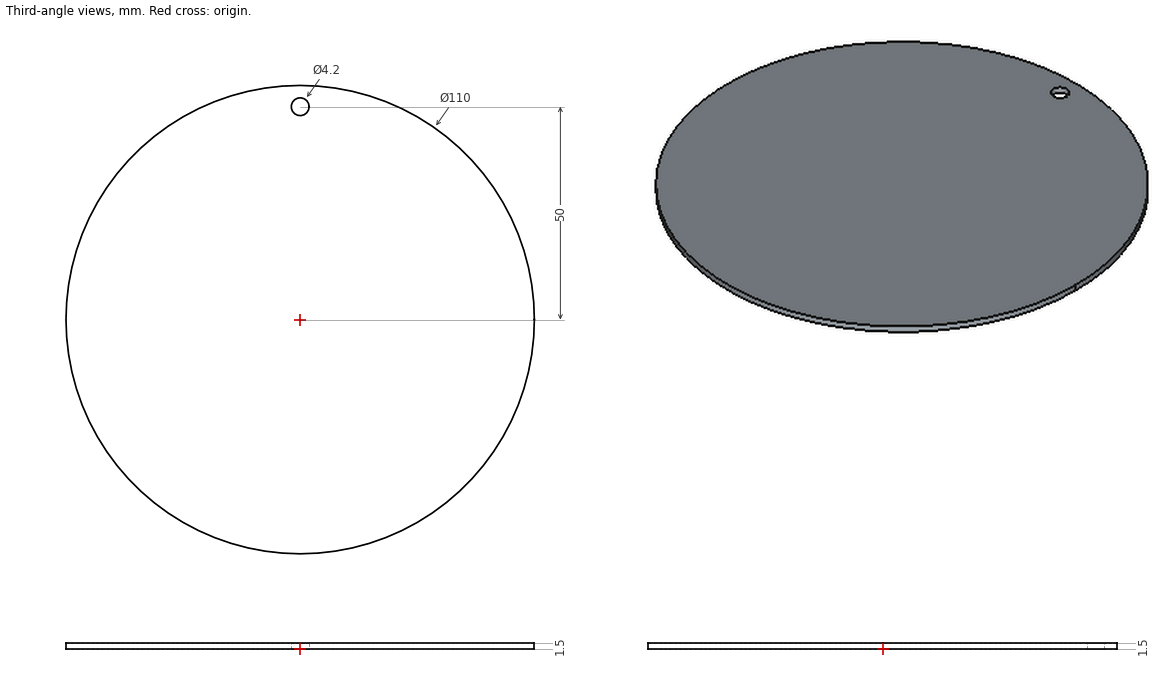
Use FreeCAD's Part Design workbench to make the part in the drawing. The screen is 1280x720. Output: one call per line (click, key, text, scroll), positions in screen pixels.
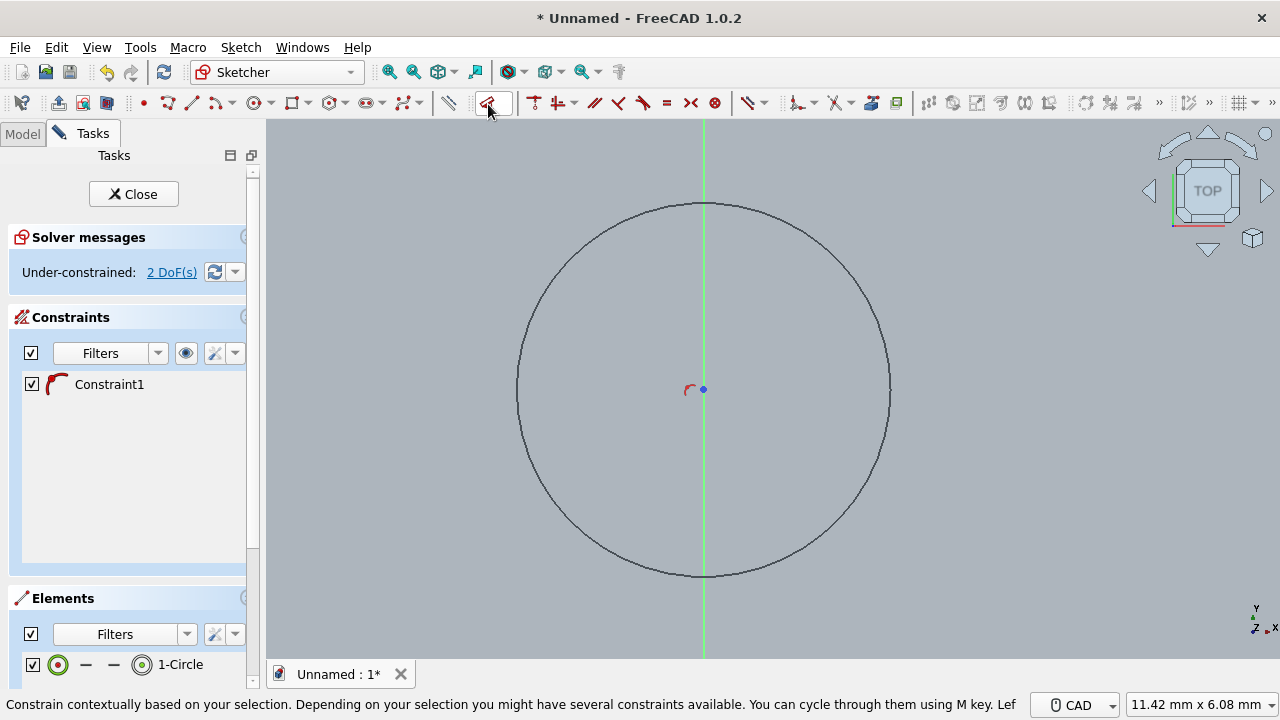
click(835, 257)
click(857, 234)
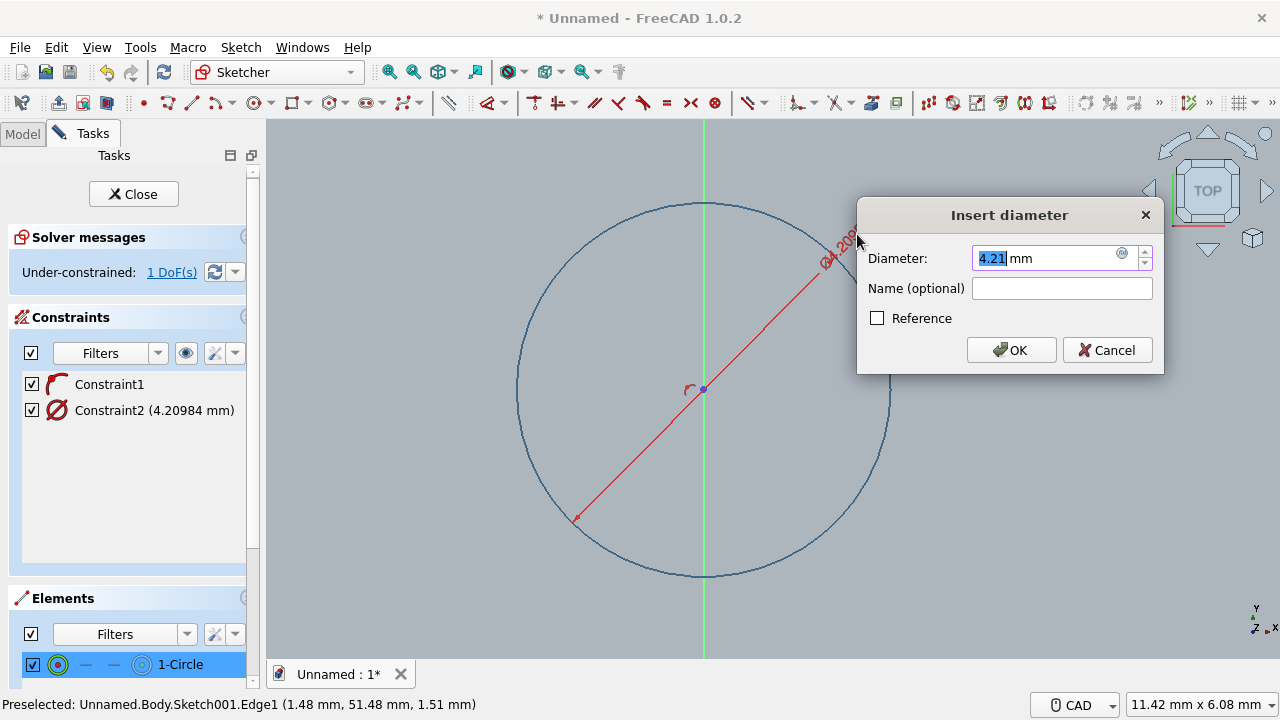
text(4.2)
key(Return)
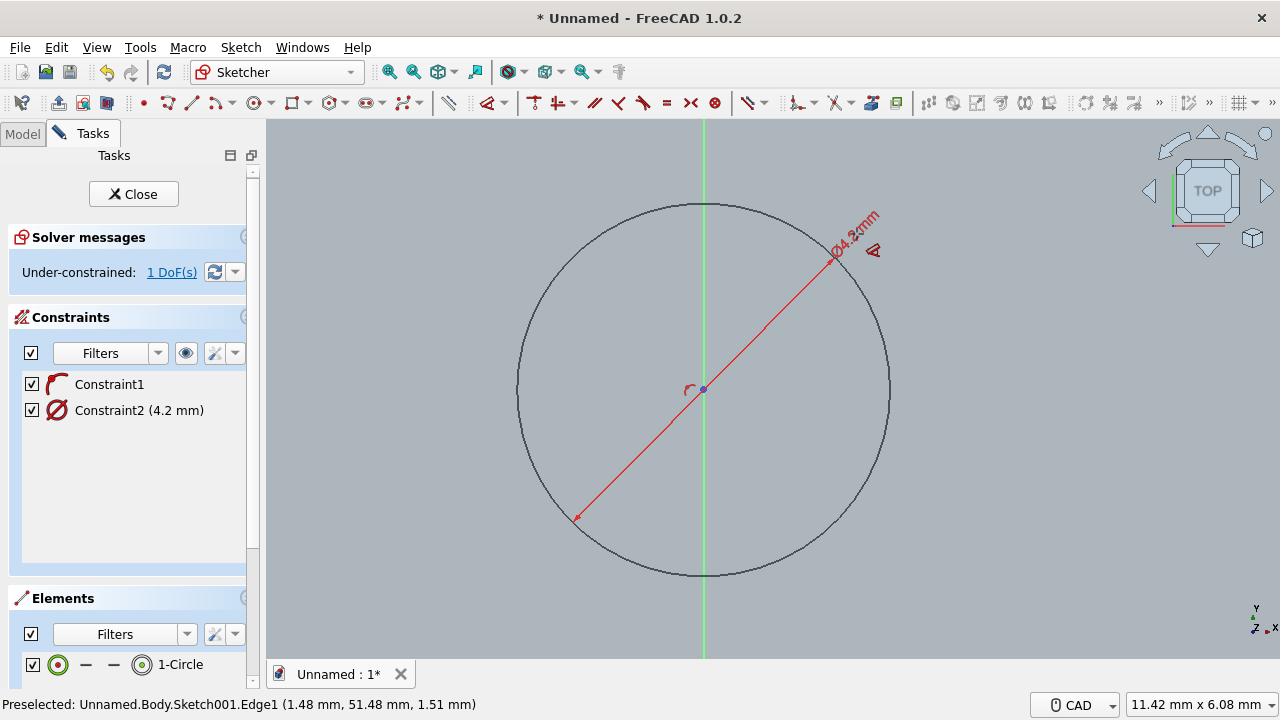
click(704, 390)
click(738, 510)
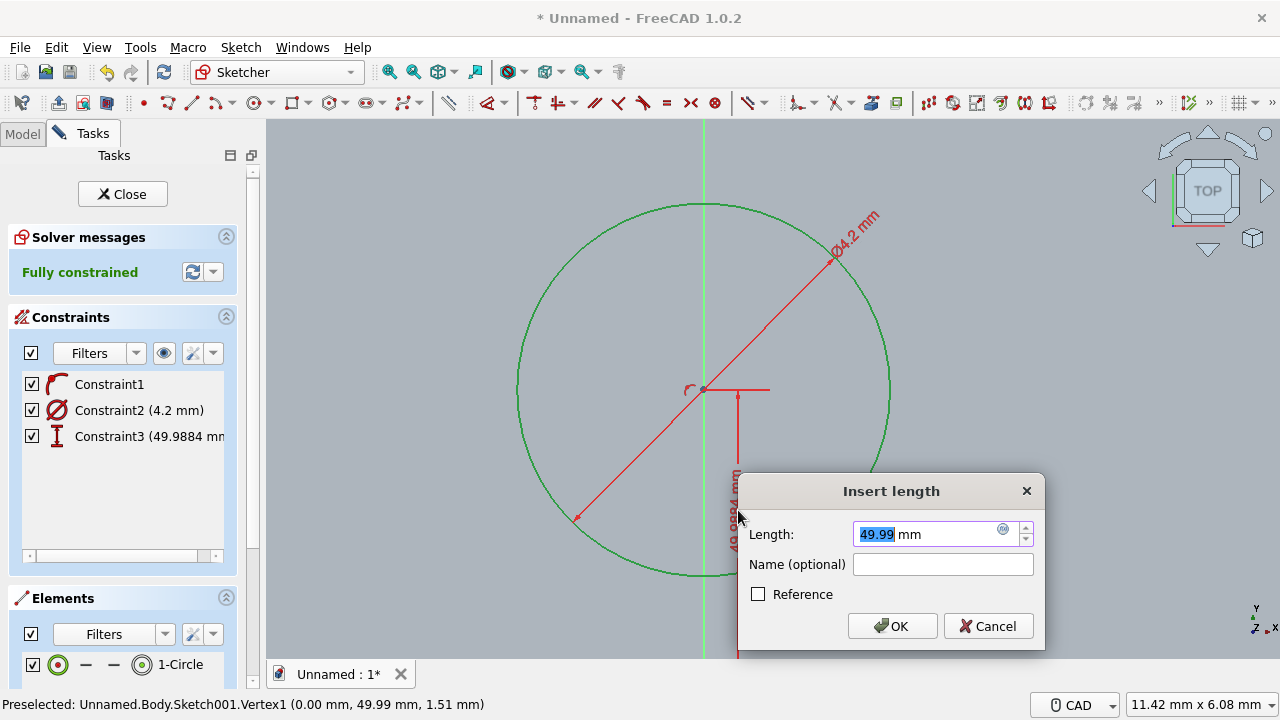
text(50)
key(Return)
key(Escape)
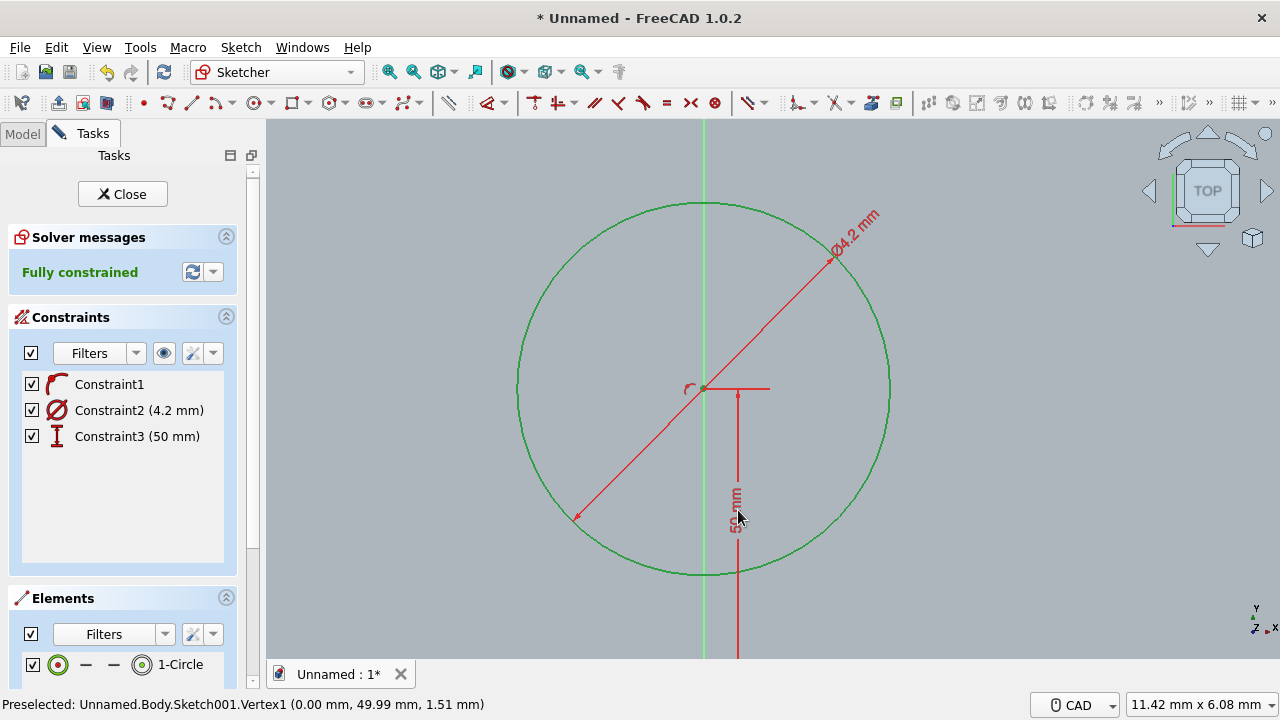
click(123, 194)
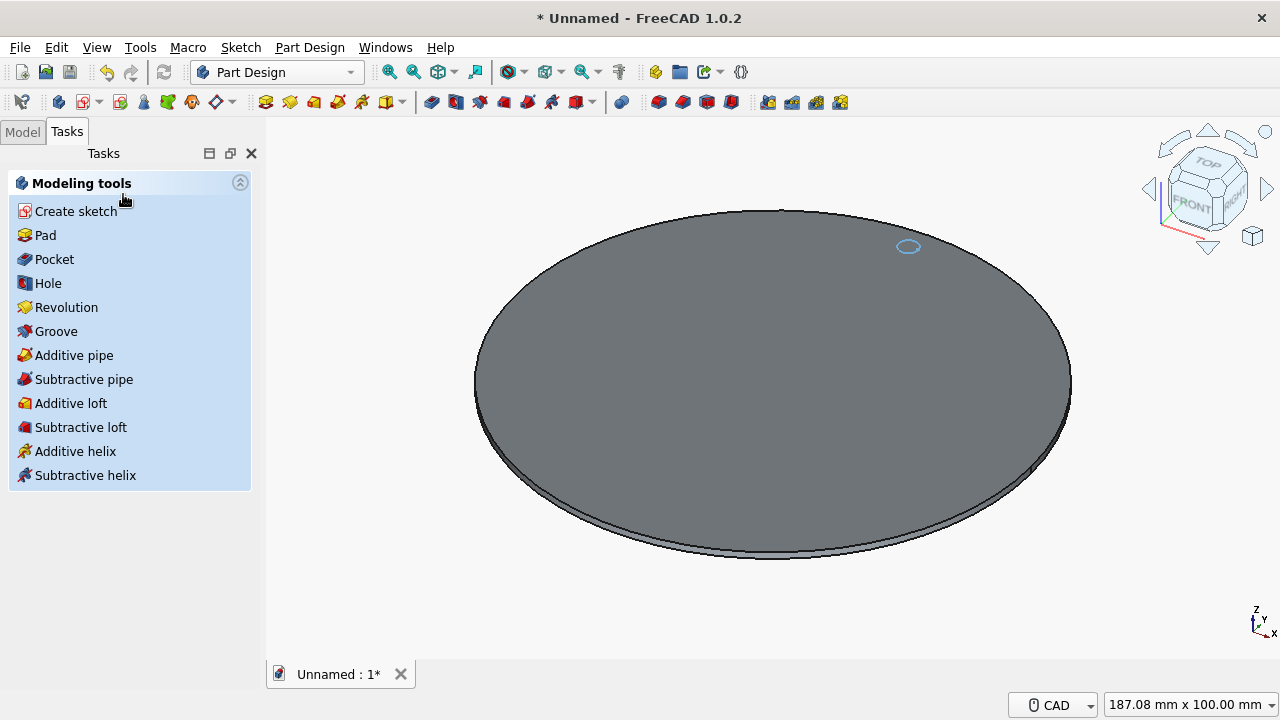
click(432, 102)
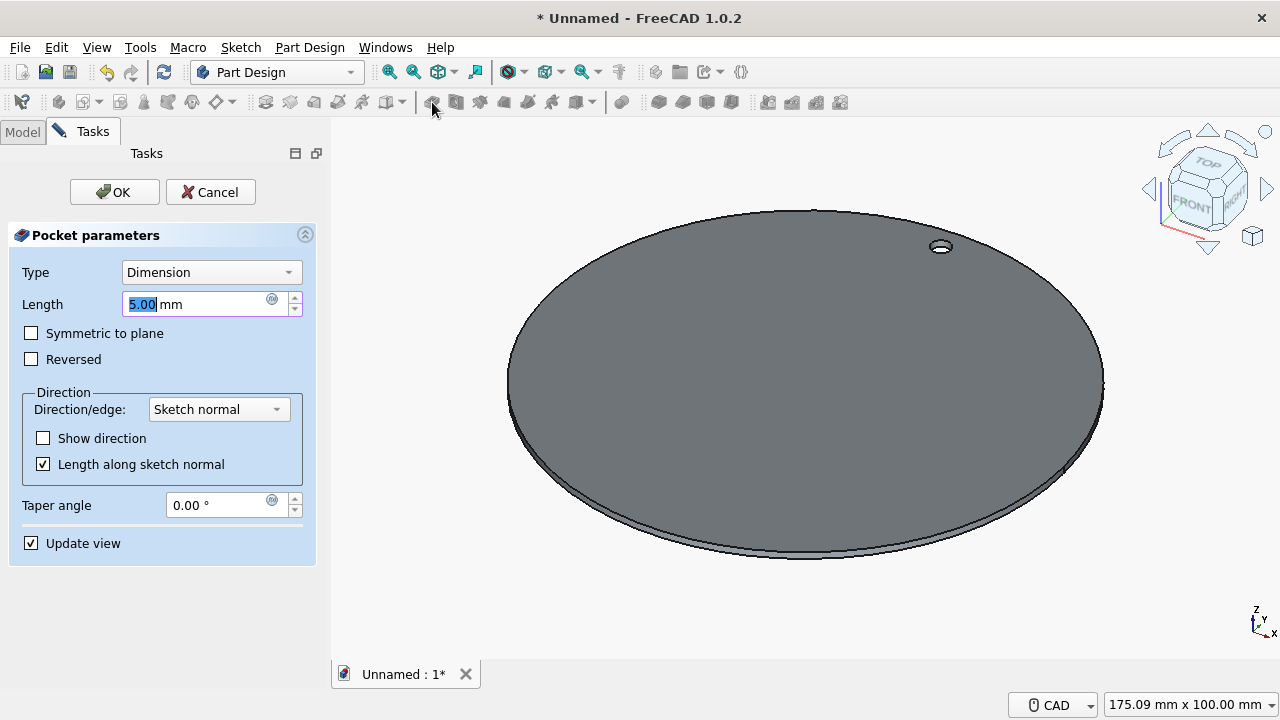
text(1.5)
key(Tab)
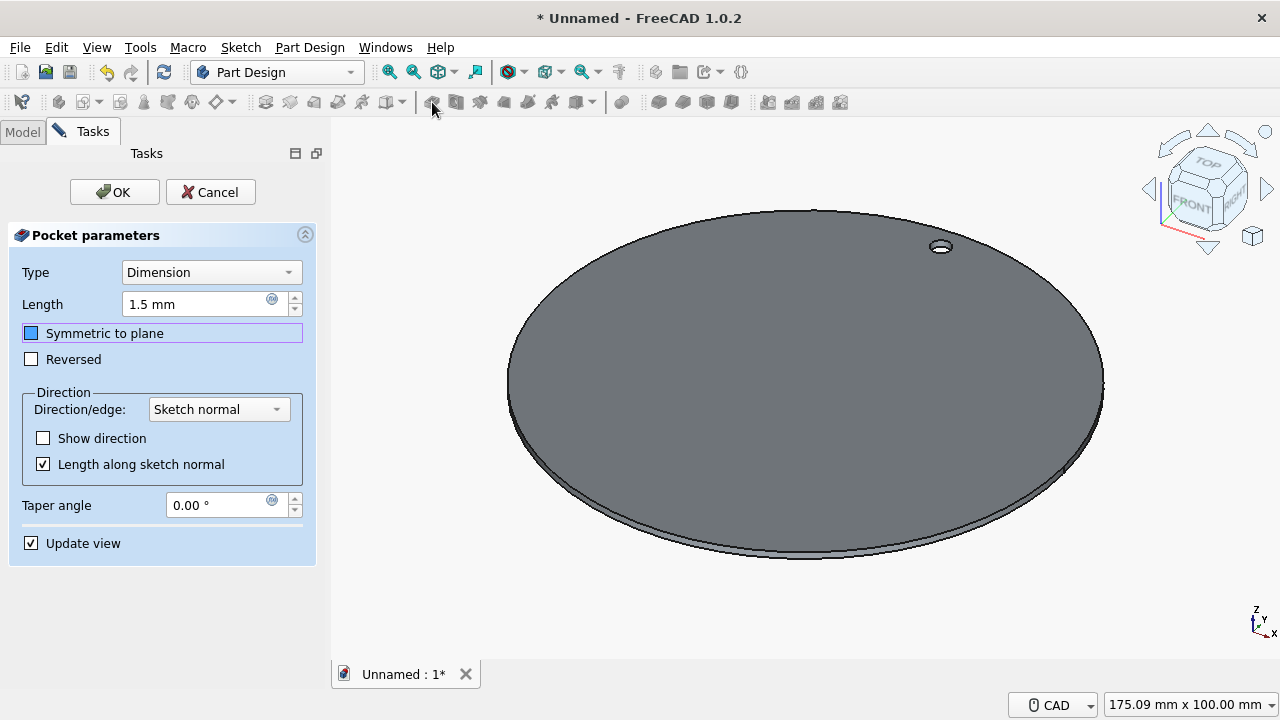
click(115, 192)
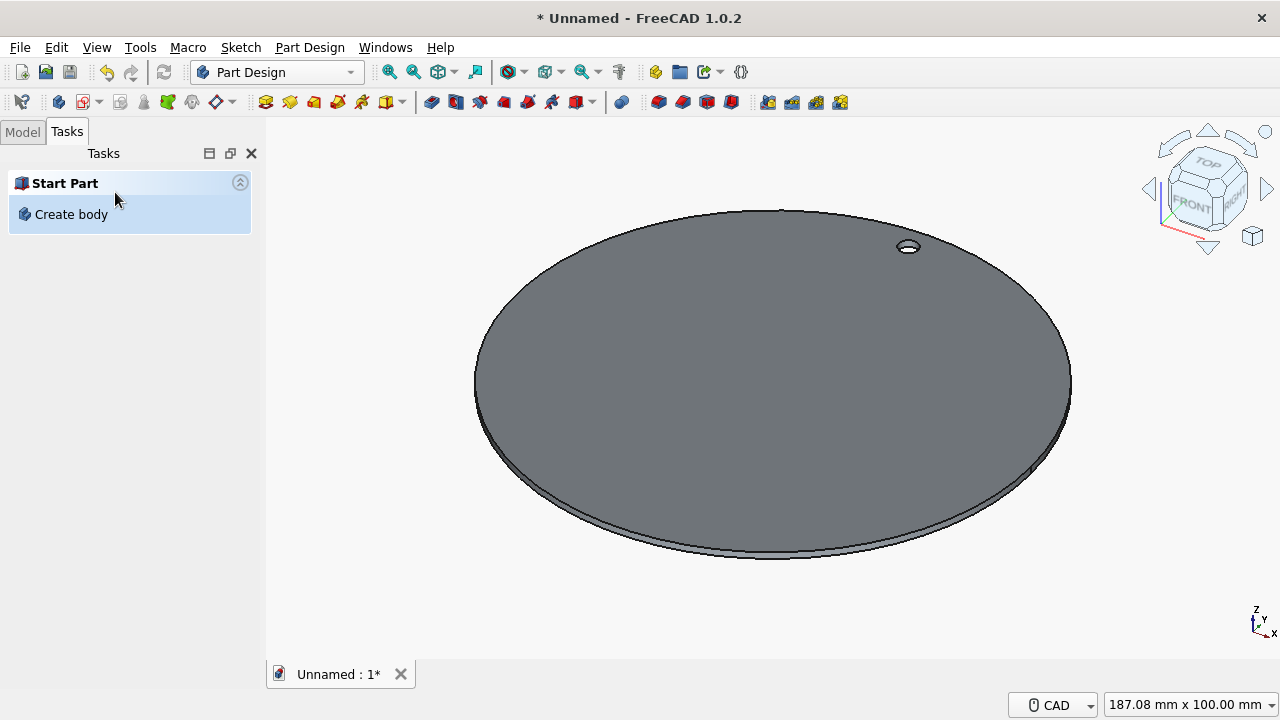
key(0)